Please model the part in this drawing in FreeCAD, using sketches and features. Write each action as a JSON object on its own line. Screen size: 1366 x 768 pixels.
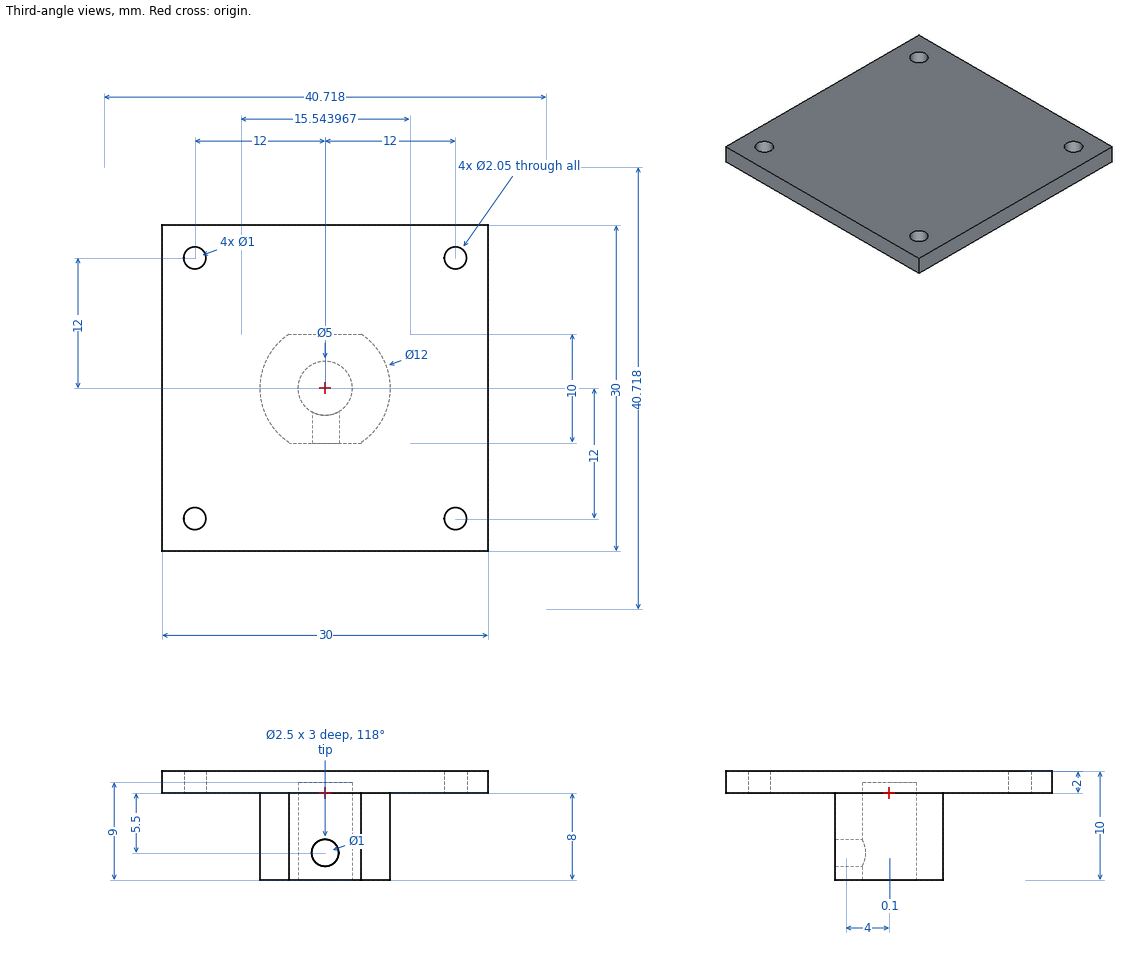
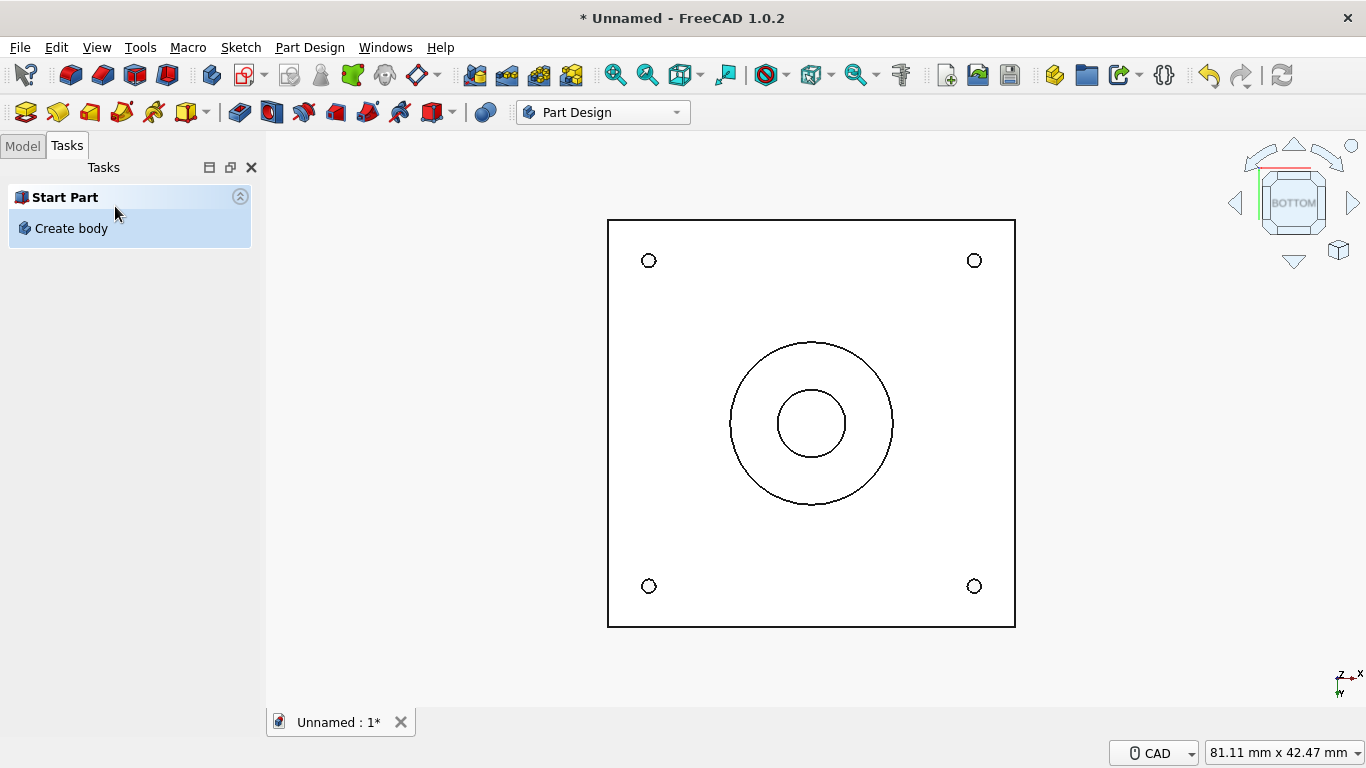
{"action": "left_click", "coordinate": [788, 469]}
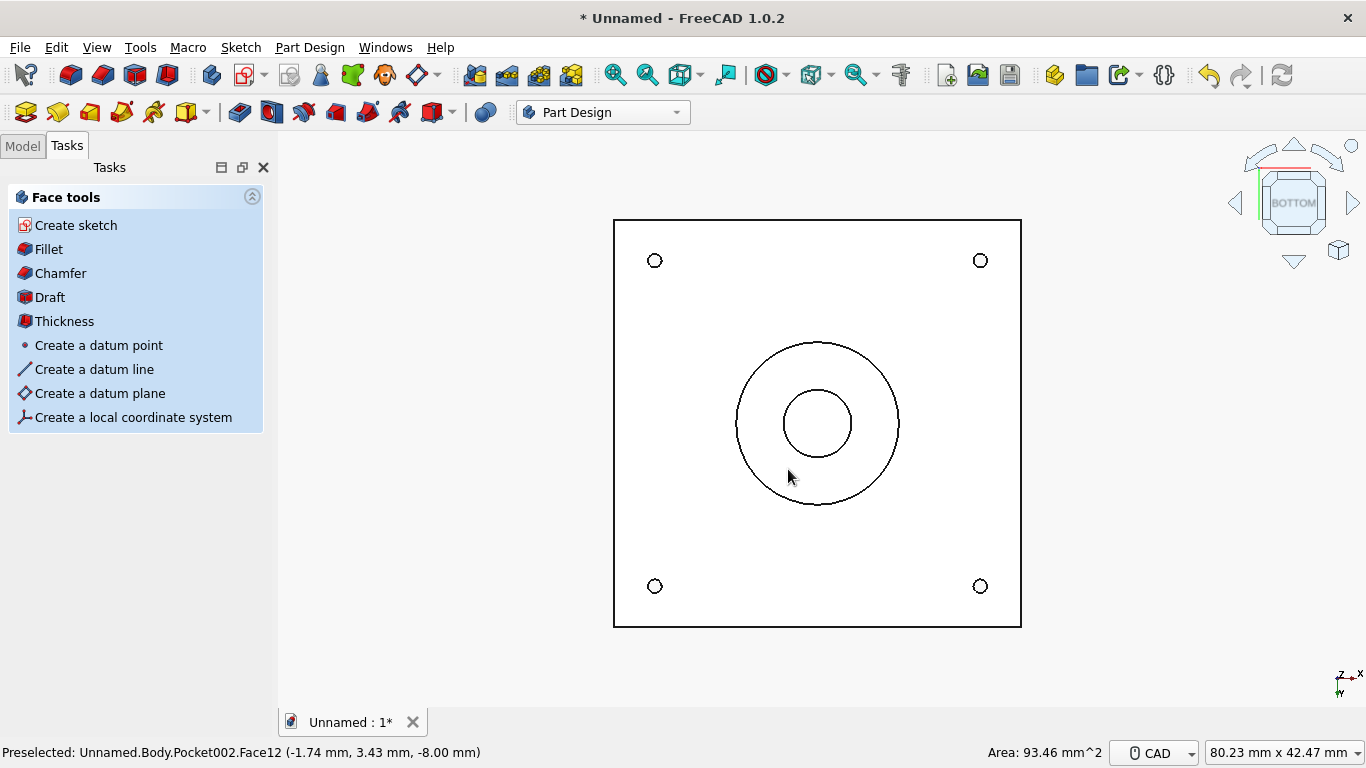
{"action": "left_click", "coordinate": [244, 76]}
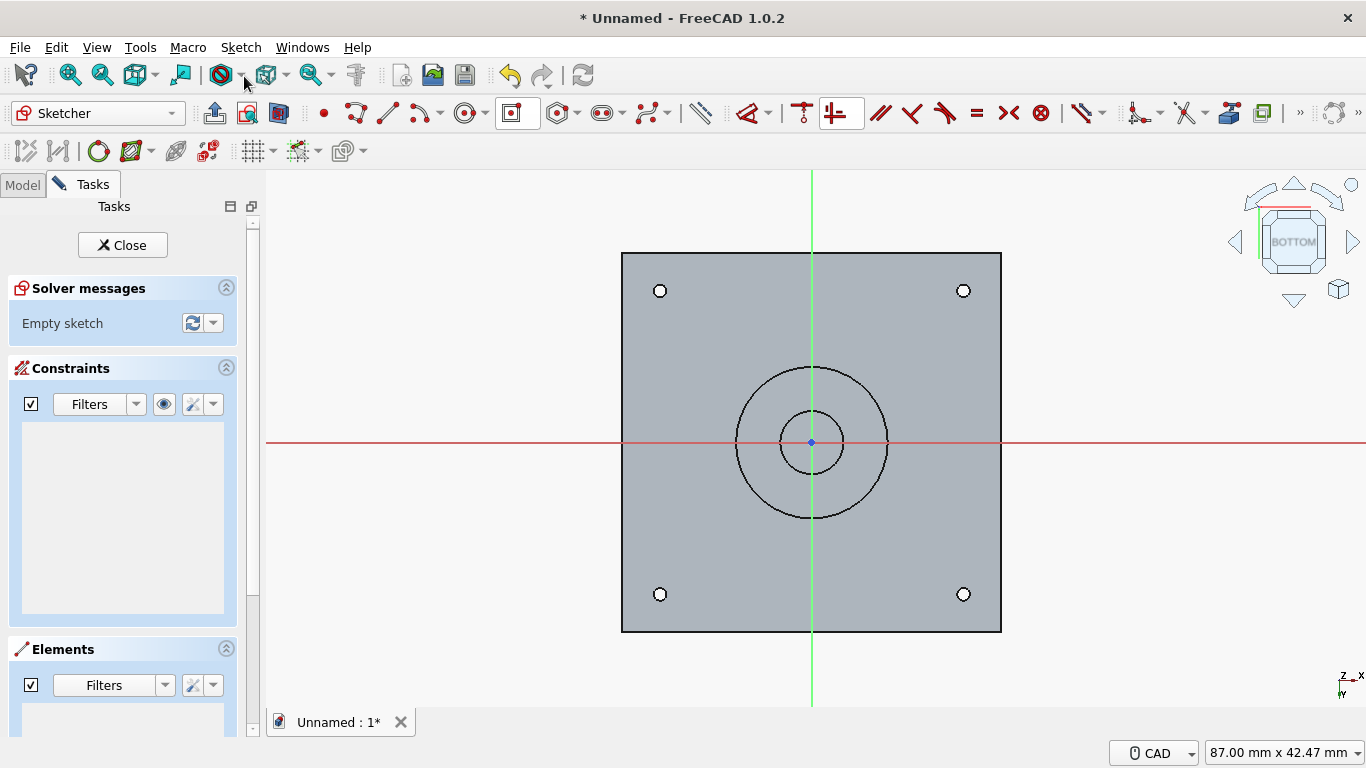
{"action": "scroll", "coordinate": [617, 430], "scroll_direction": "down", "scroll_amount": 2}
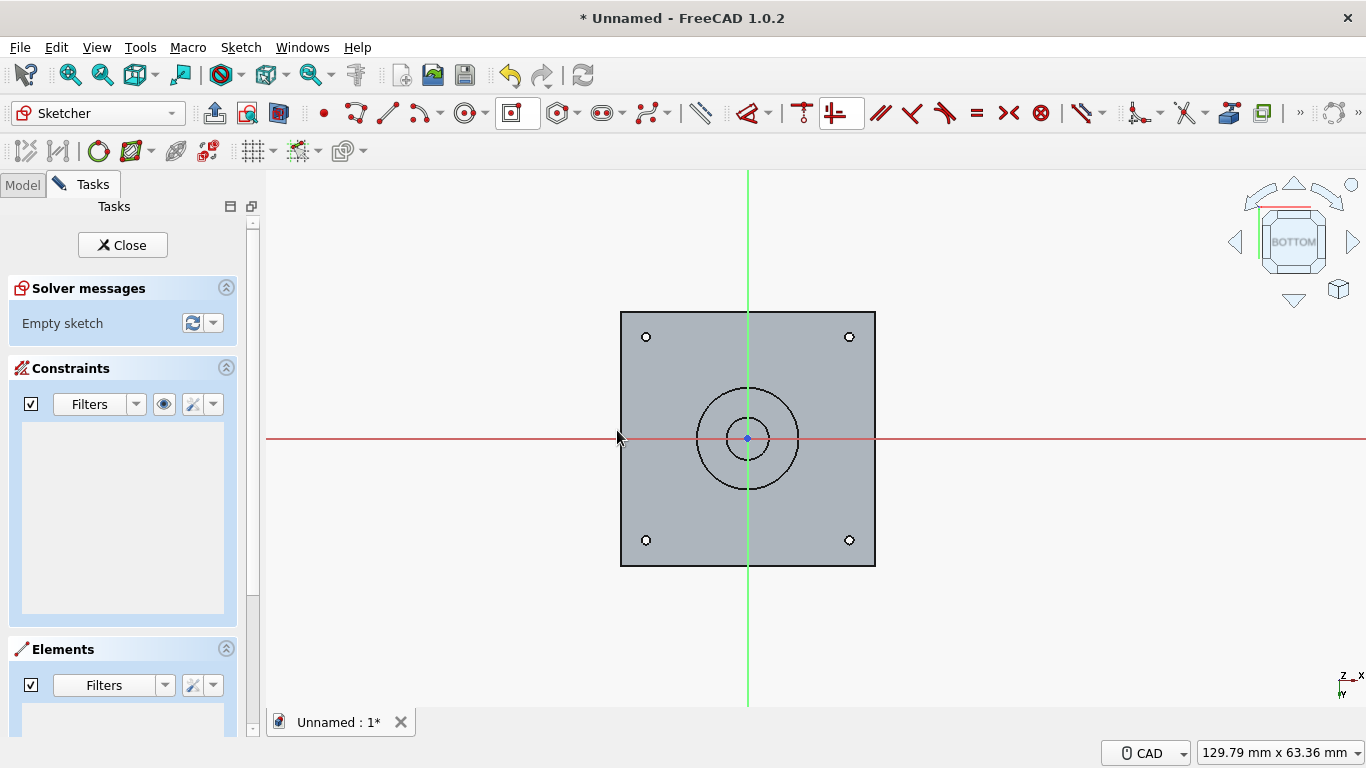
{"action": "left_click", "coordinate": [512, 114]}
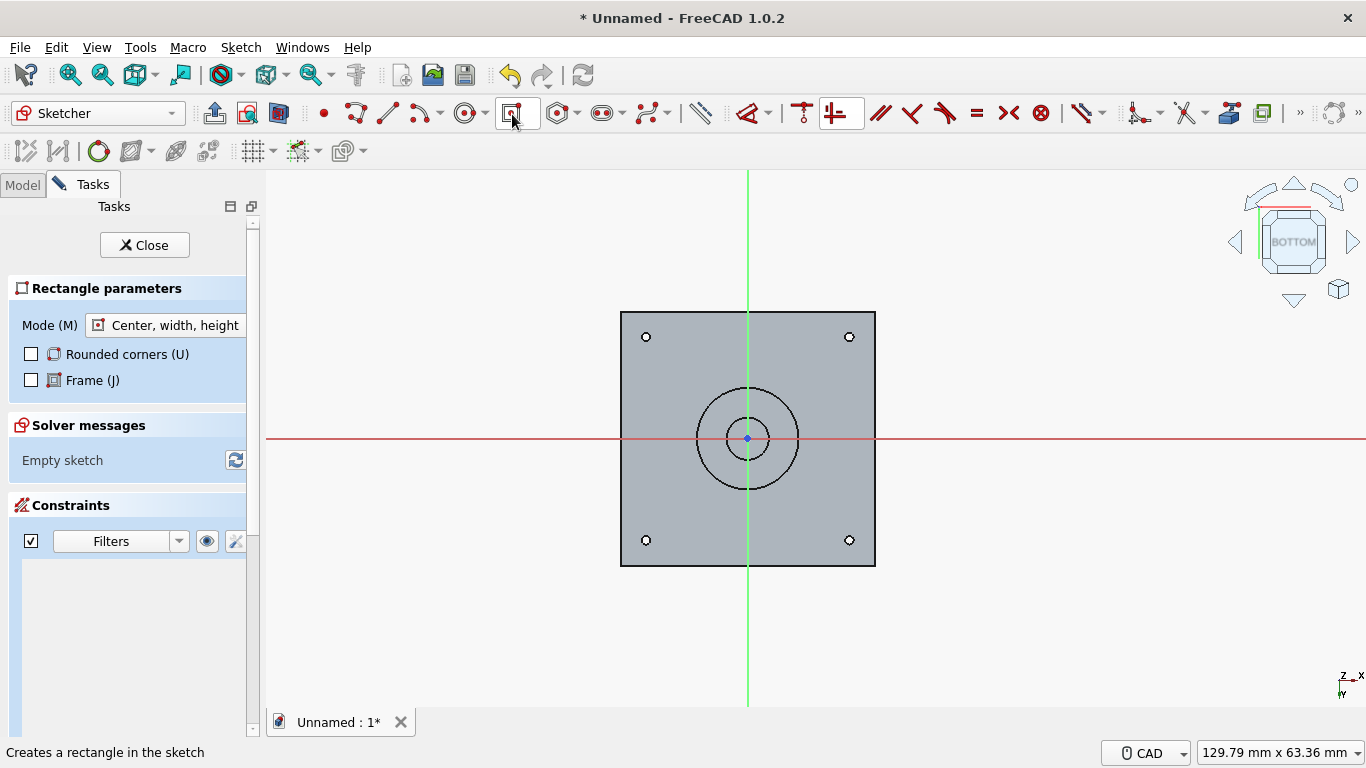
{"action": "left_click", "coordinate": [748, 439]}
{"action": "left_click", "coordinate": [920, 266]}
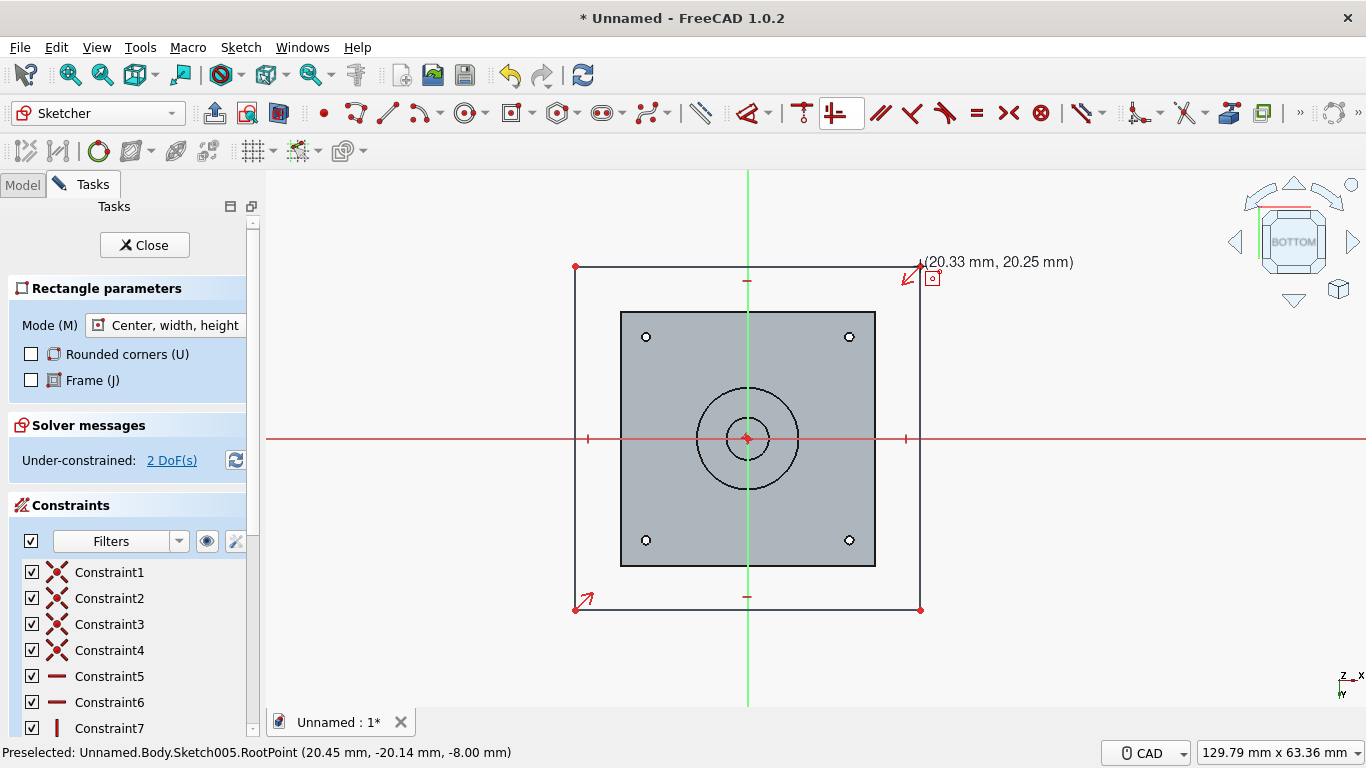
{"action": "left_click", "coordinate": [748, 439]}
{"action": "left_click", "coordinate": [814, 396]}
{"action": "key", "text": "Escape"}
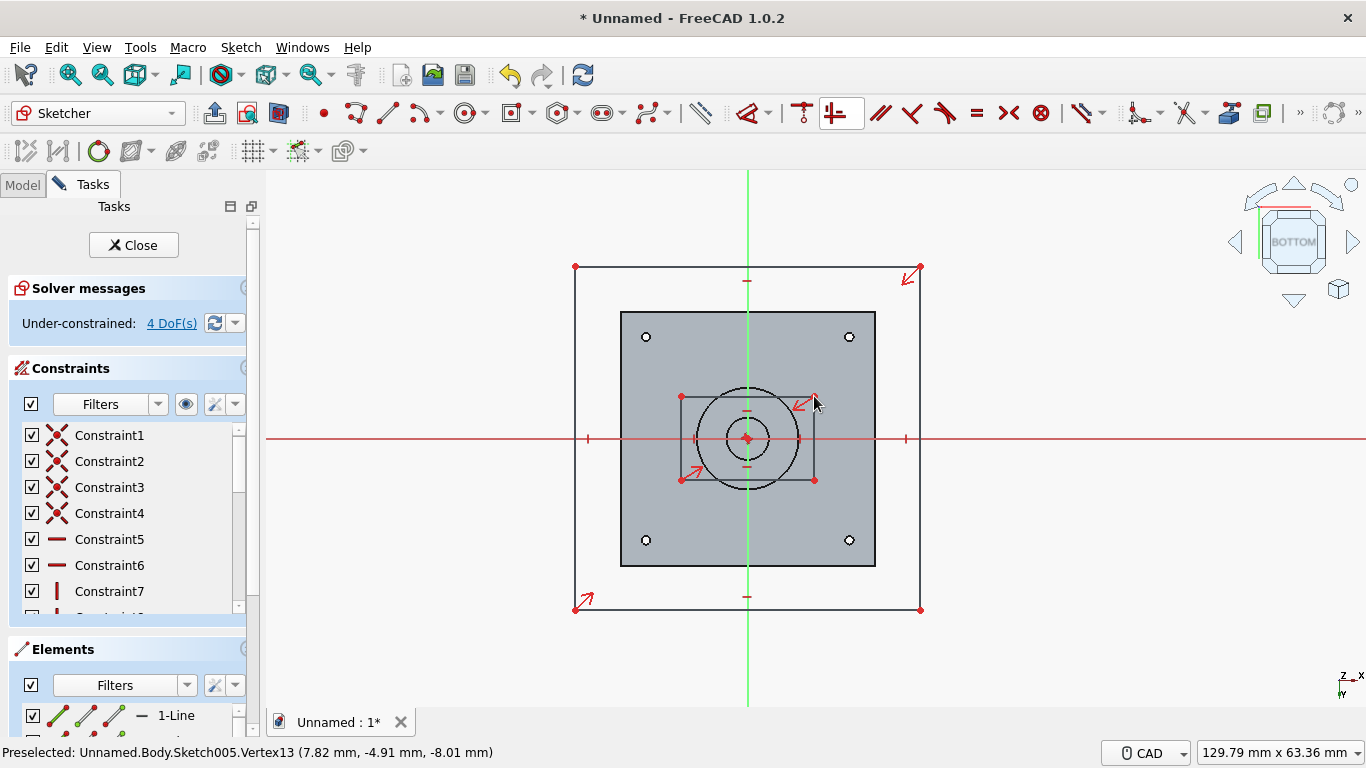
{"action": "left_click", "coordinate": [748, 114]}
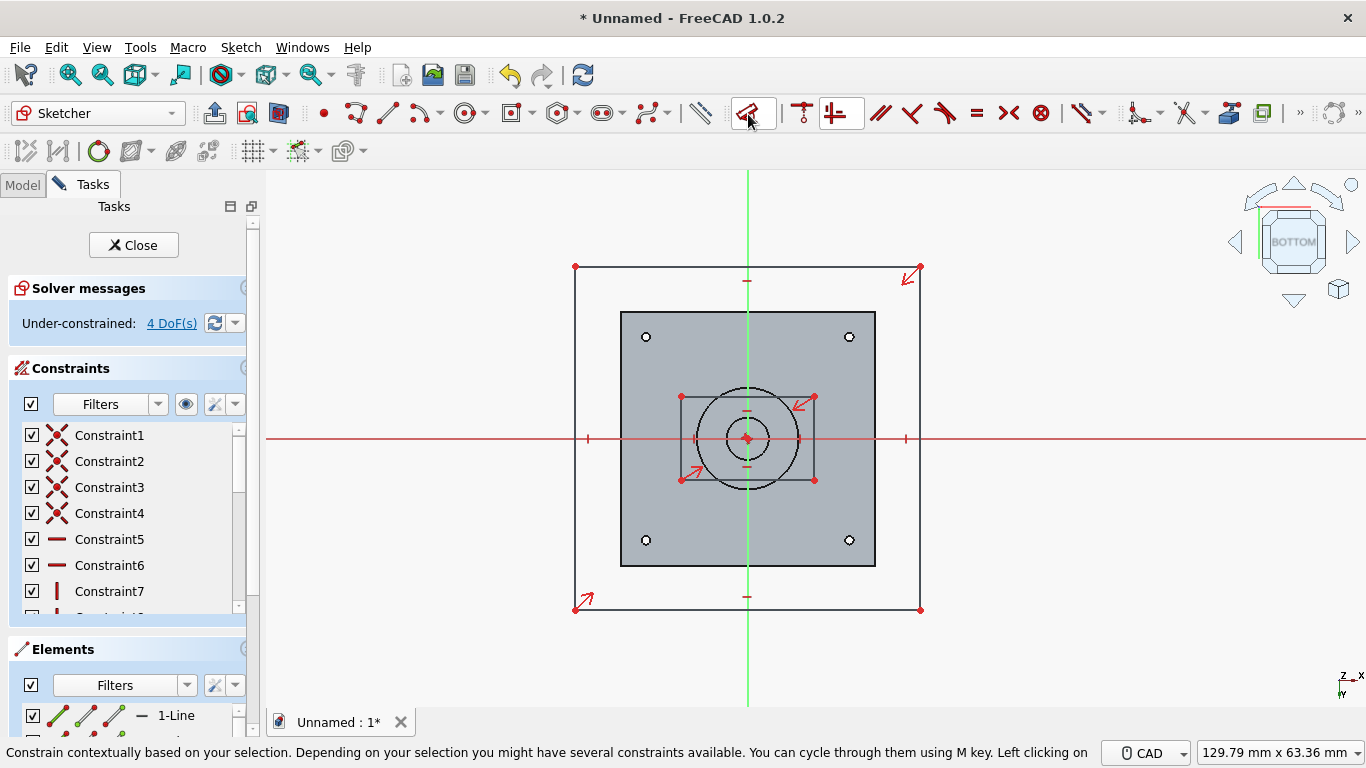
{"action": "left_click", "coordinate": [814, 455]}
{"action": "left_click", "coordinate": [848, 419]}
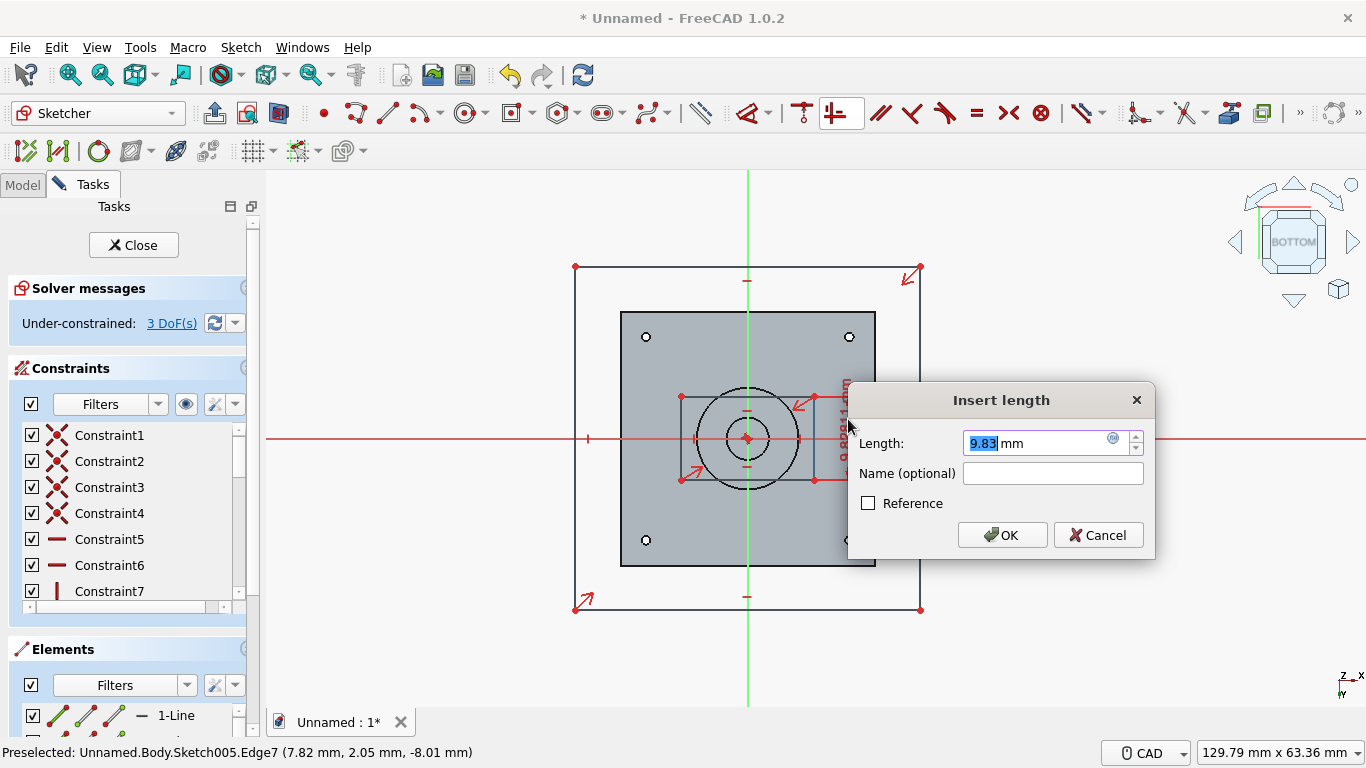
{"action": "type", "text": "10"}
{"action": "key", "text": "Return"}